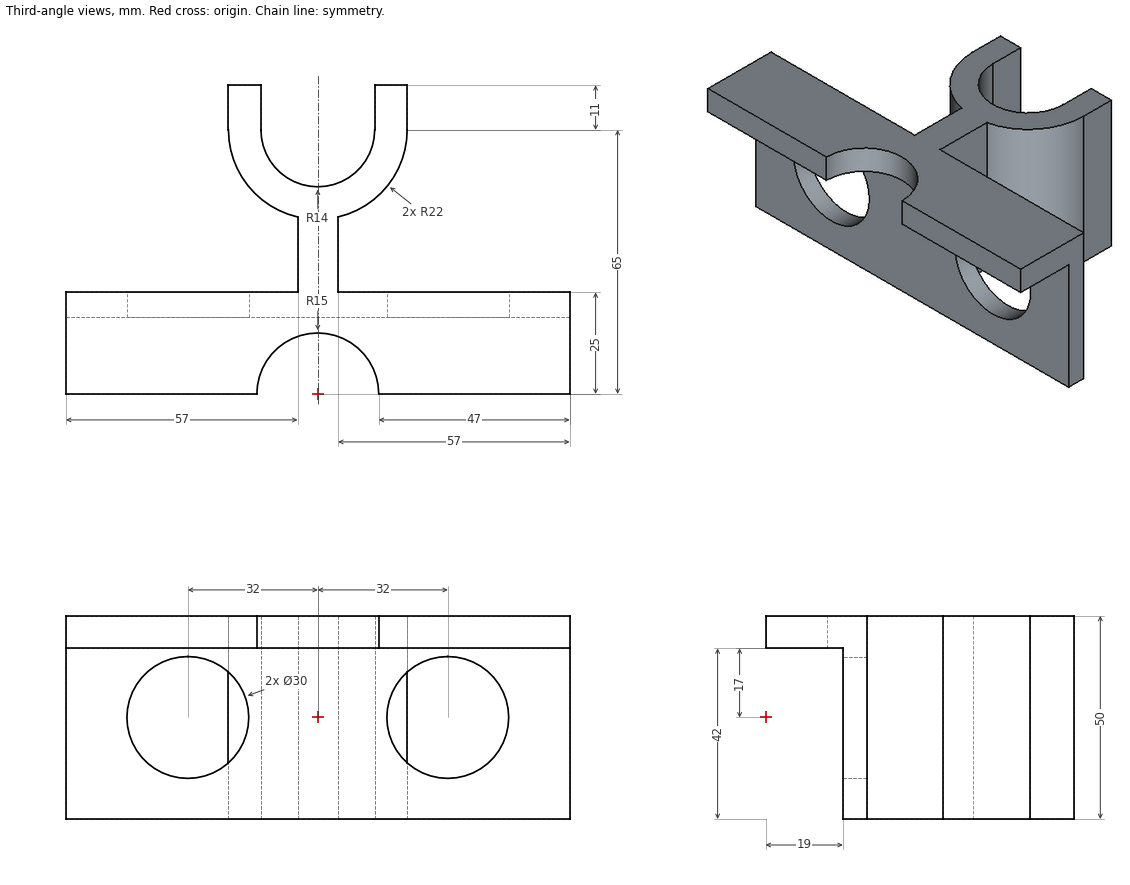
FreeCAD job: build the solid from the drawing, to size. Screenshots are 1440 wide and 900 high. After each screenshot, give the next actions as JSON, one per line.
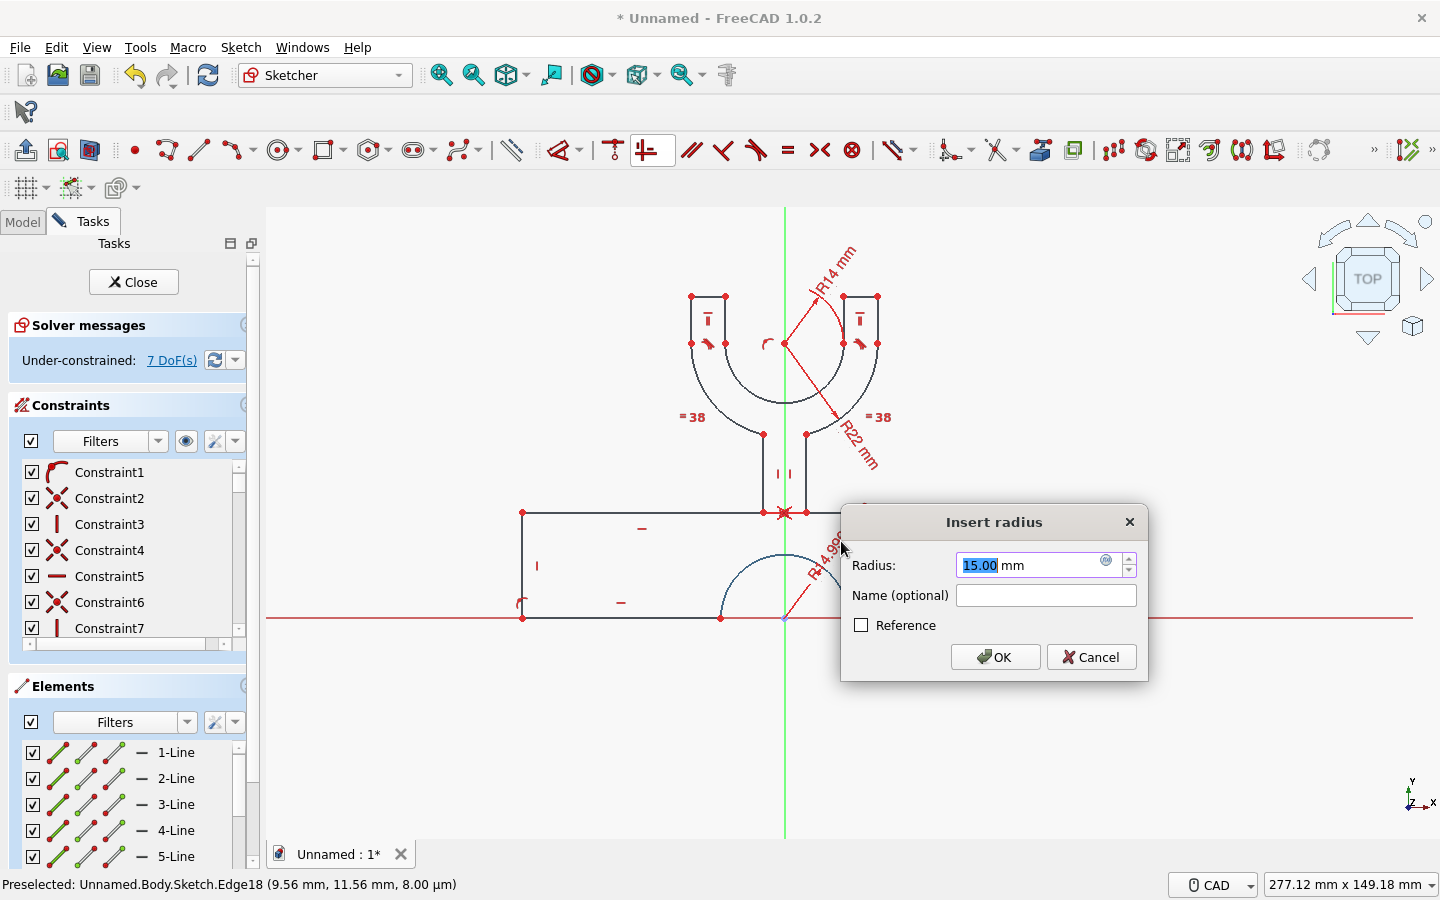
{"action": "type", "text": "15"}
{"action": "key", "text": "Return"}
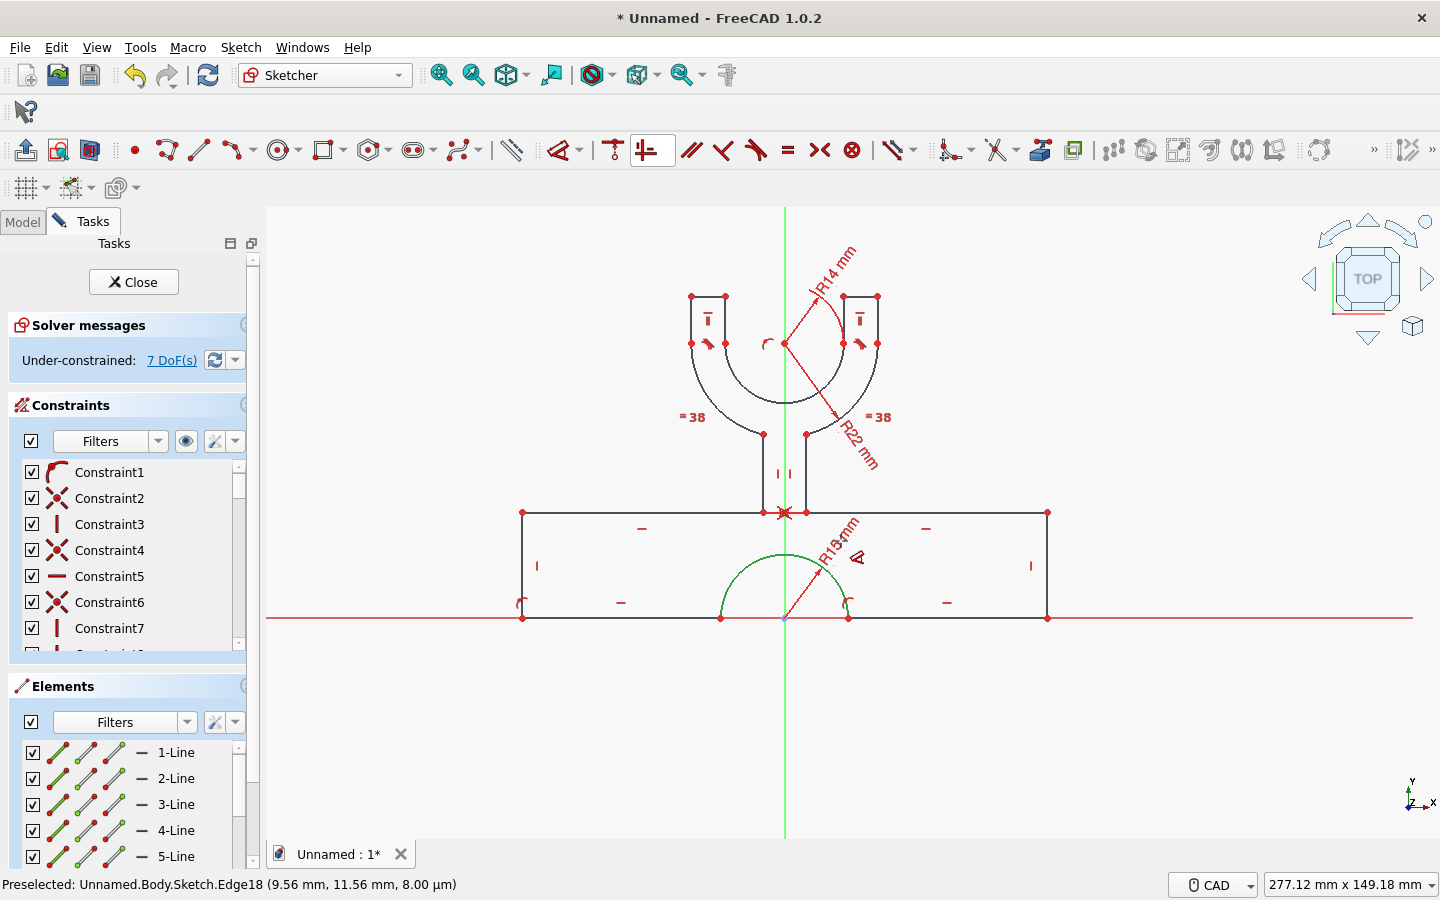
{"action": "left_click", "coordinate": [908, 618]}
{"action": "left_click", "coordinate": [948, 652]}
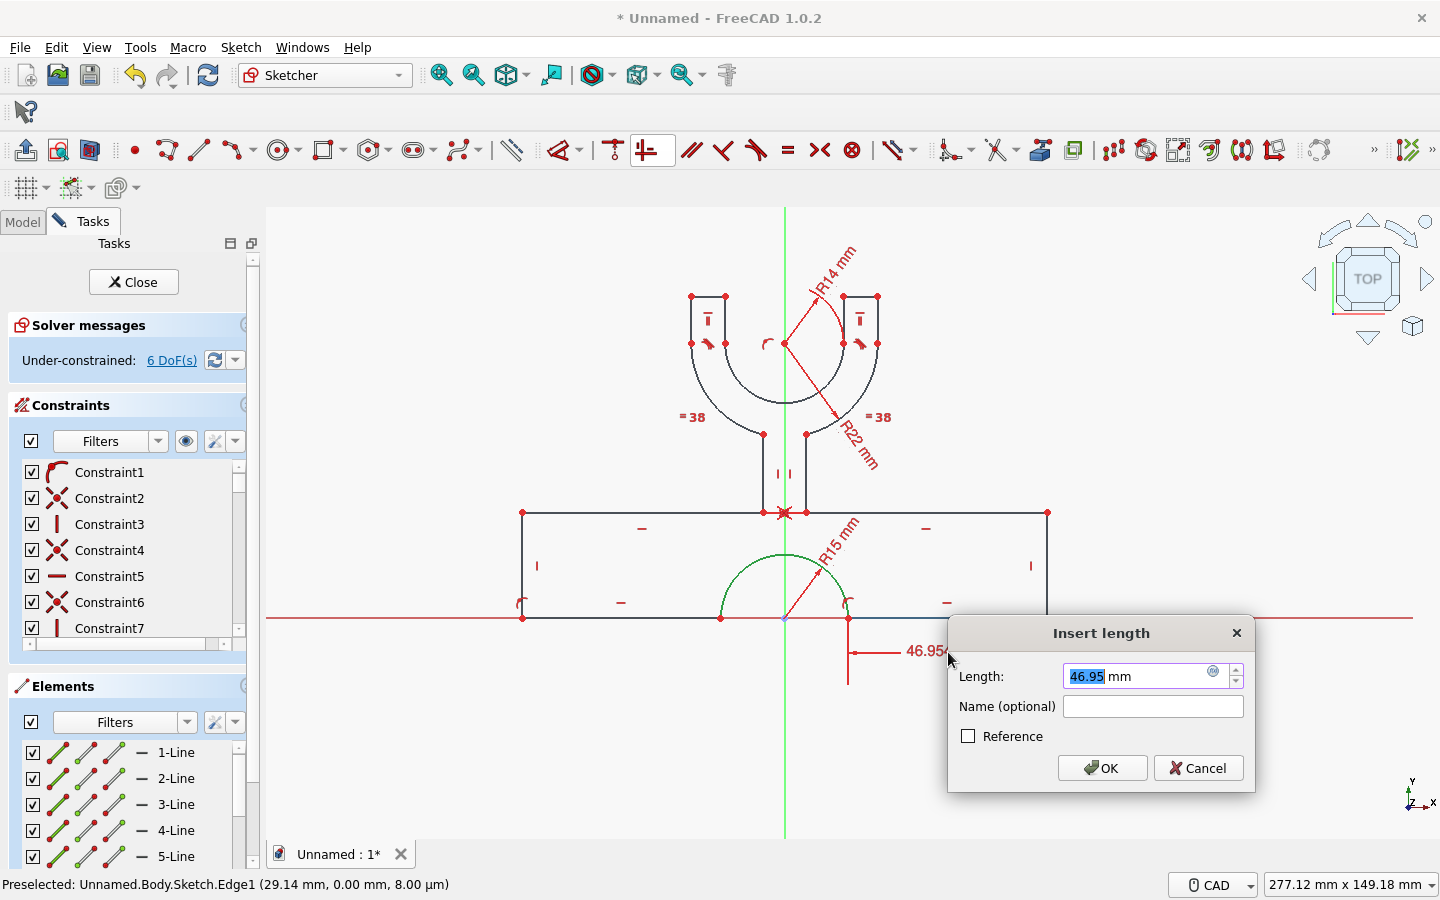
{"action": "type", "text": "47"}
{"action": "key", "text": "Return"}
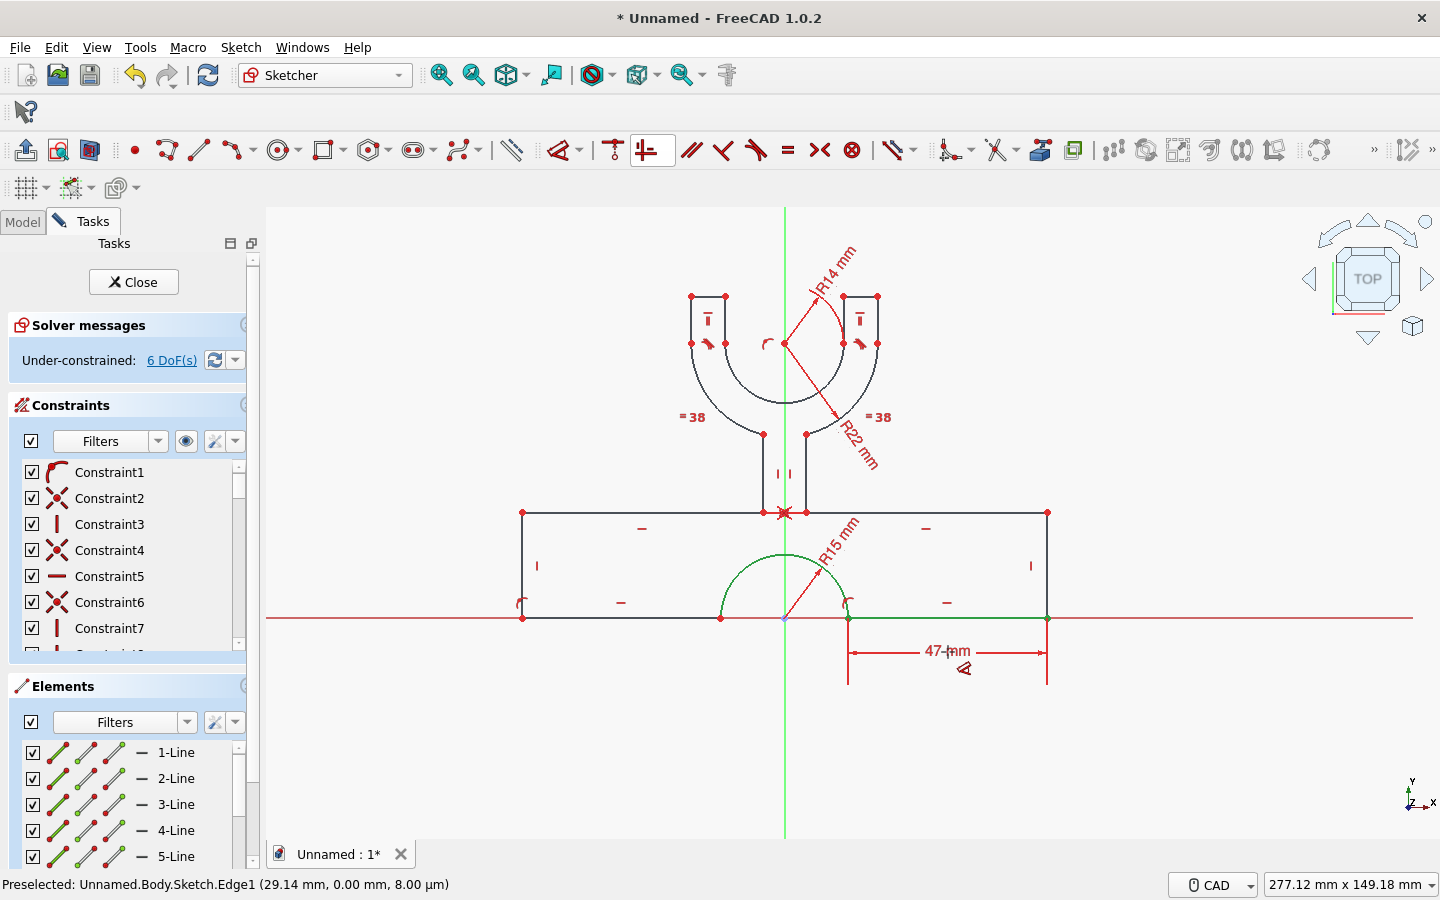
{"action": "left_click", "coordinate": [1047, 587]}
{"action": "left_click", "coordinate": [1081, 566]}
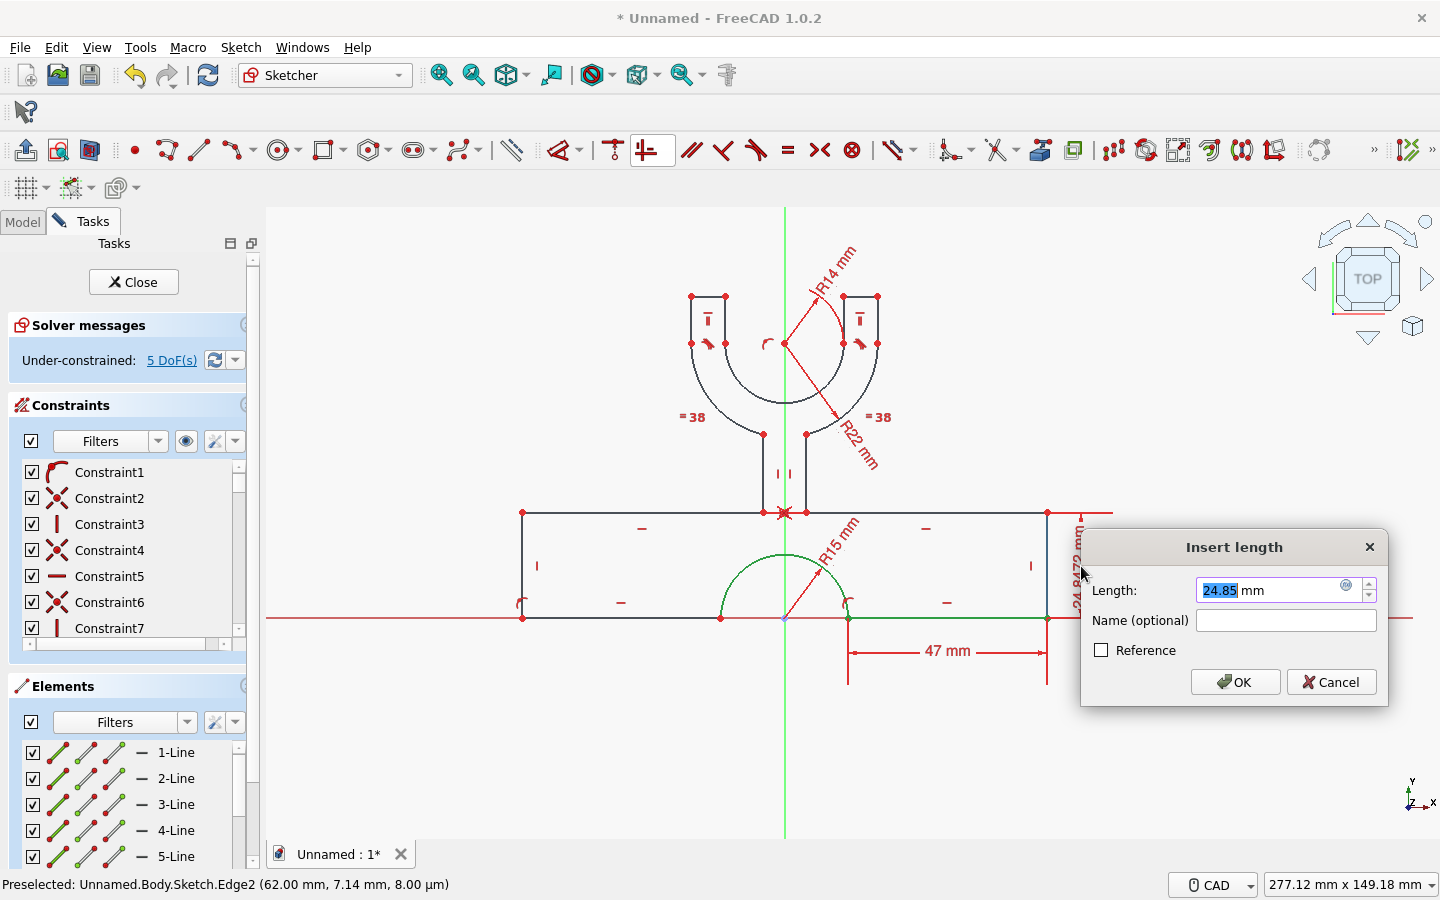
{"action": "type", "text": "25"}
{"action": "key", "text": "Return"}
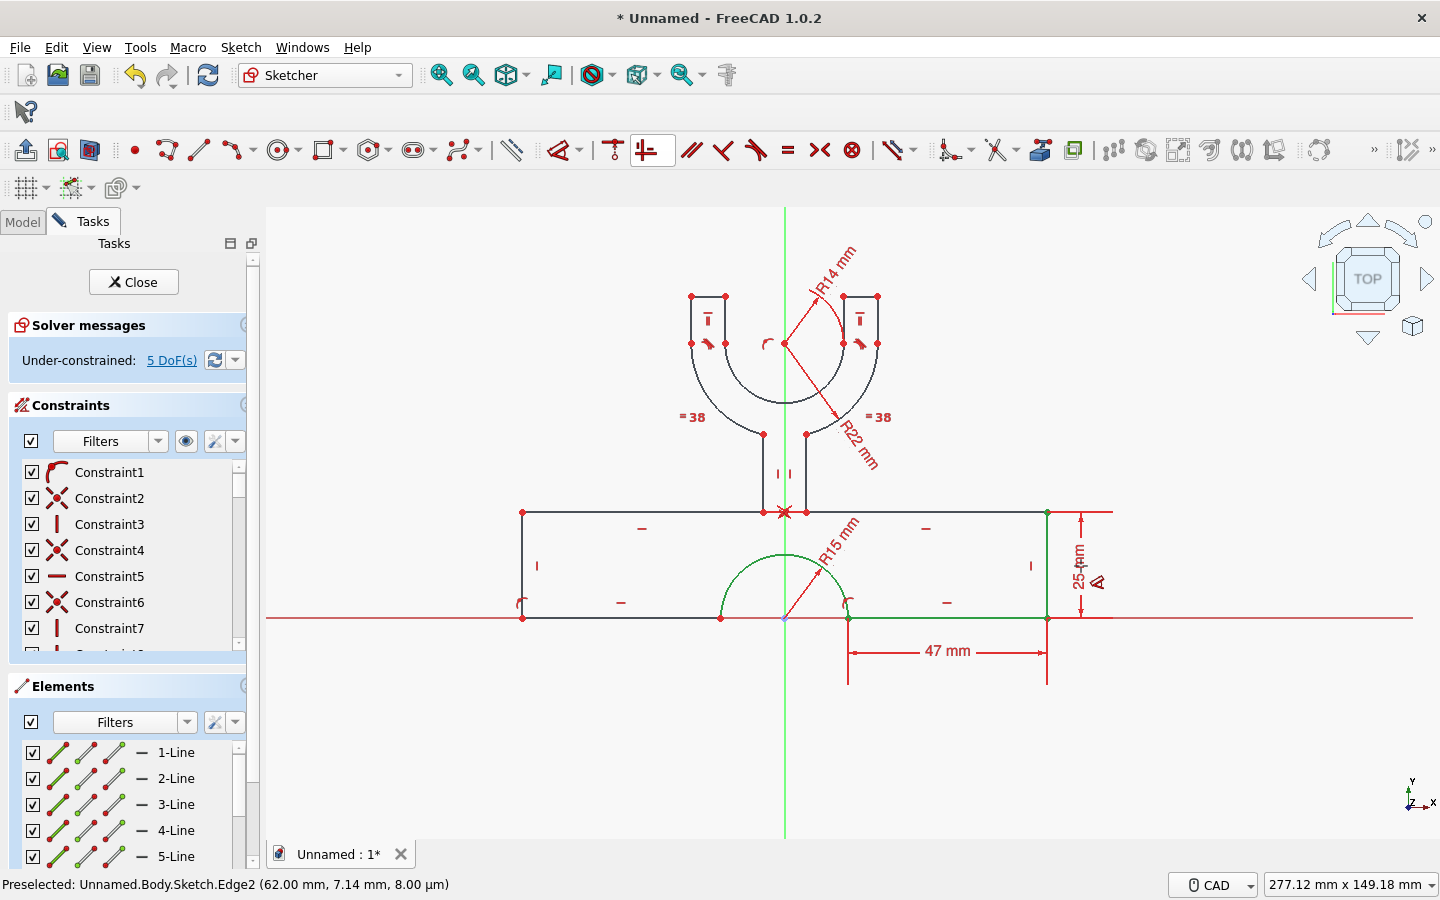
{"action": "left_click", "coordinate": [975, 512]}
{"action": "left_click", "coordinate": [927, 546]}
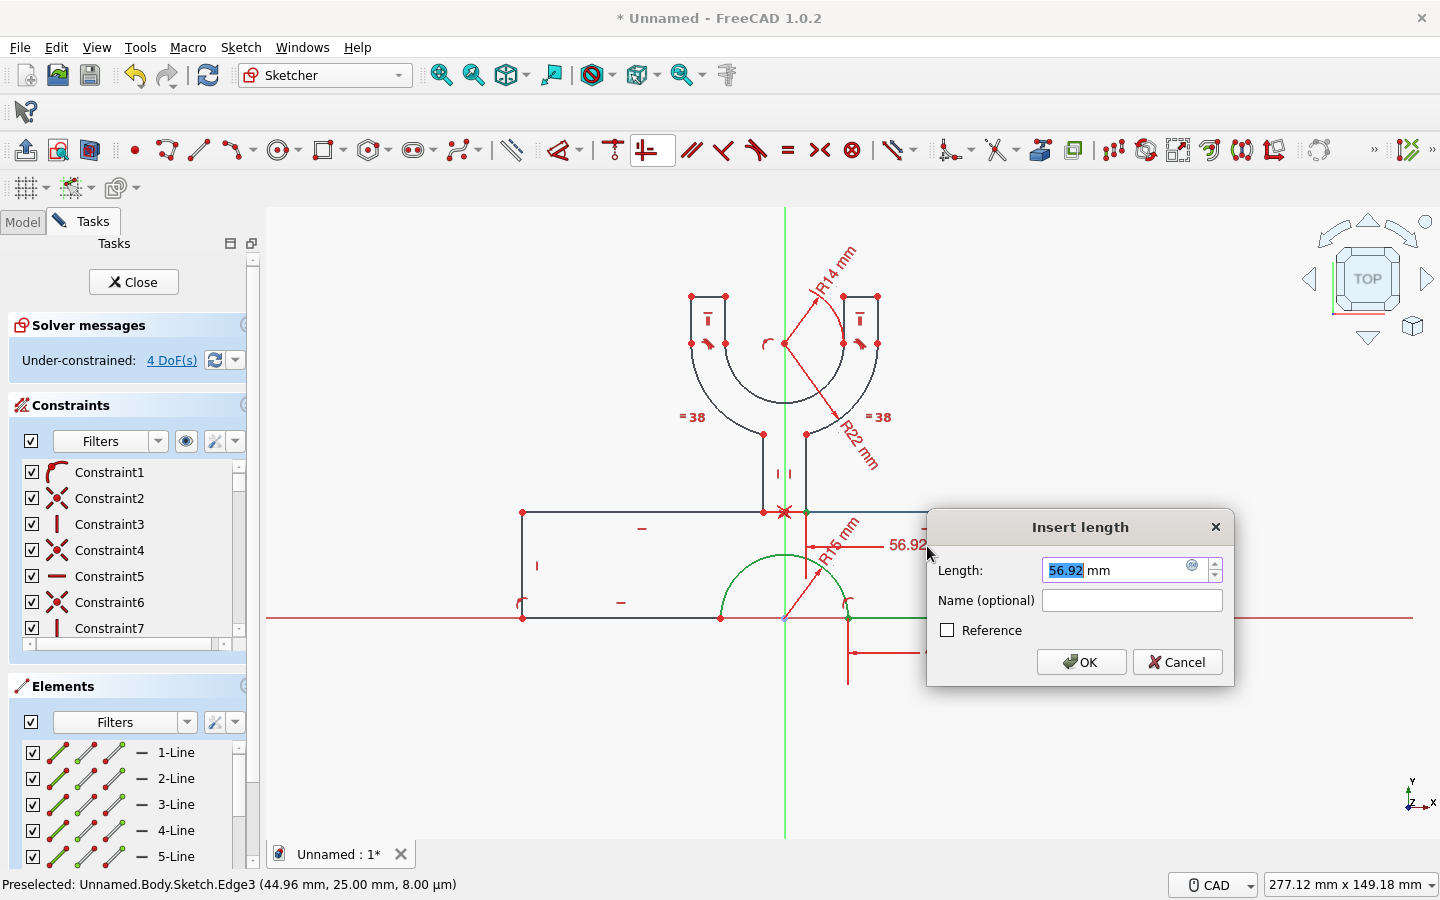
{"action": "type", "text": "57"}
{"action": "key", "text": "Return"}